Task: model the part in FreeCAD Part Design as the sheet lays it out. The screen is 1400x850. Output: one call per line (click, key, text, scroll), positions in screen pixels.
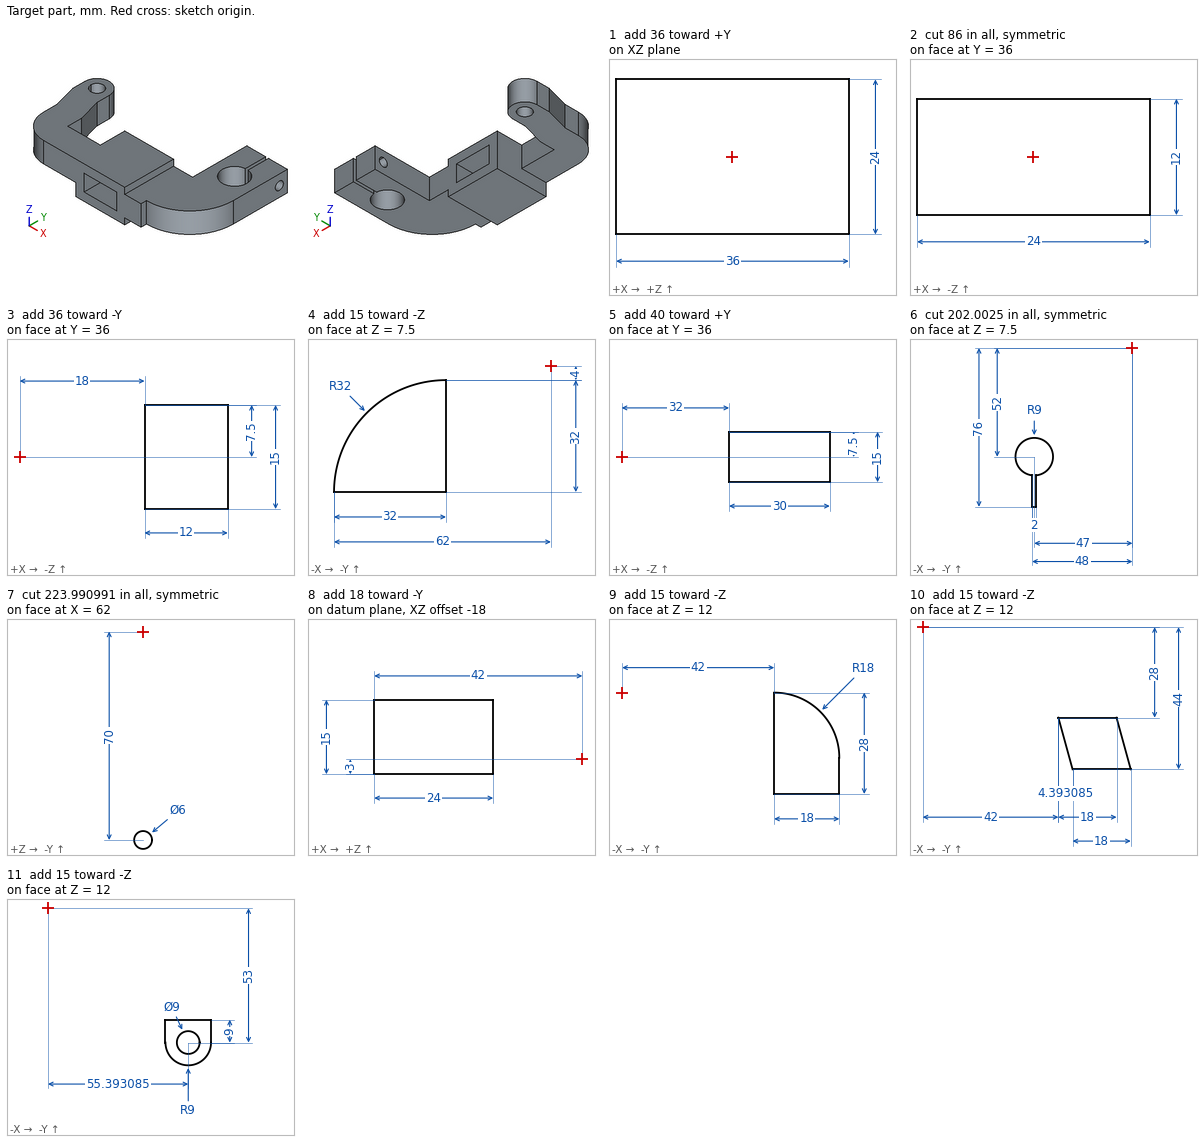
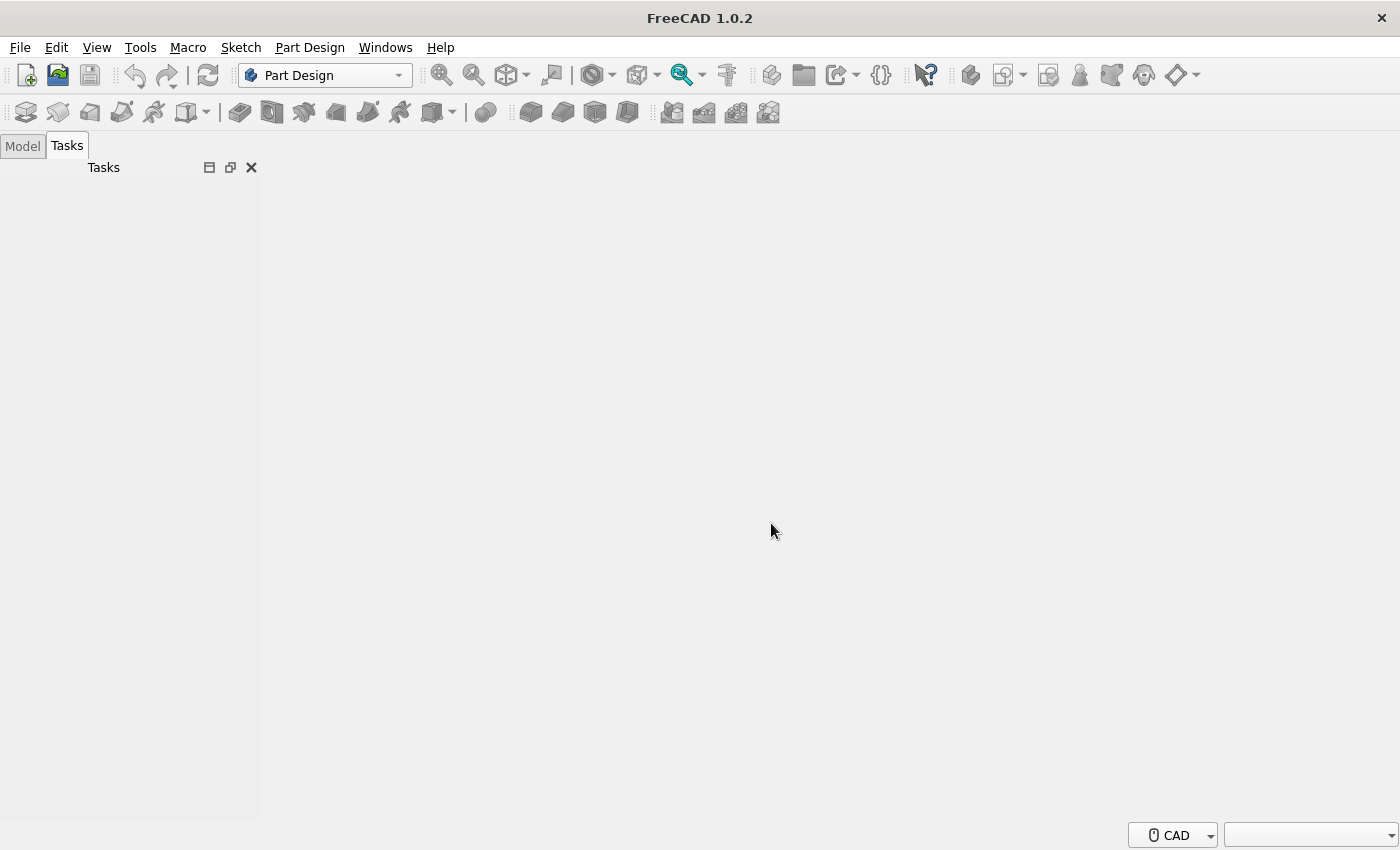
click(26, 76)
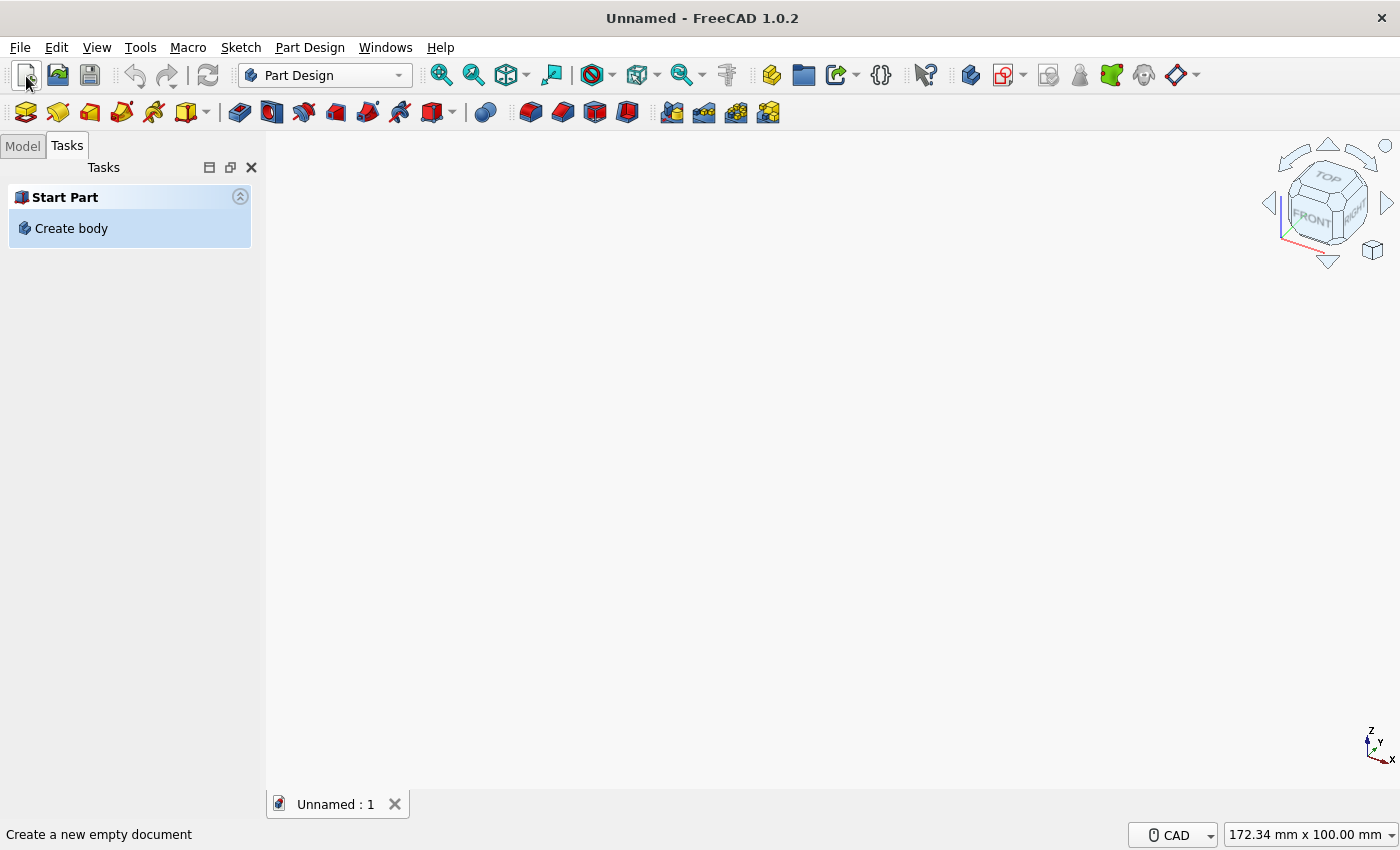
click(1004, 76)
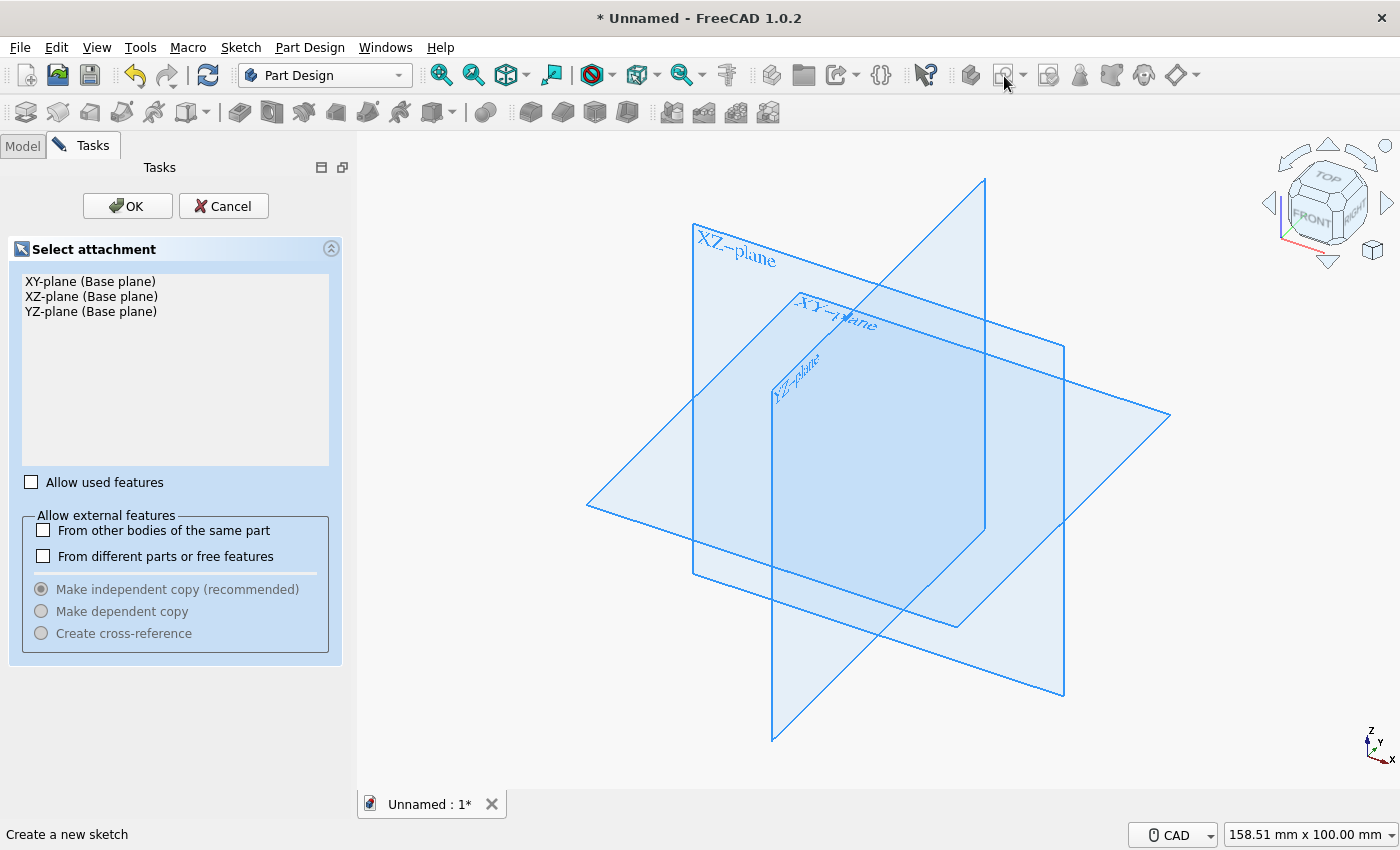
click(82, 296)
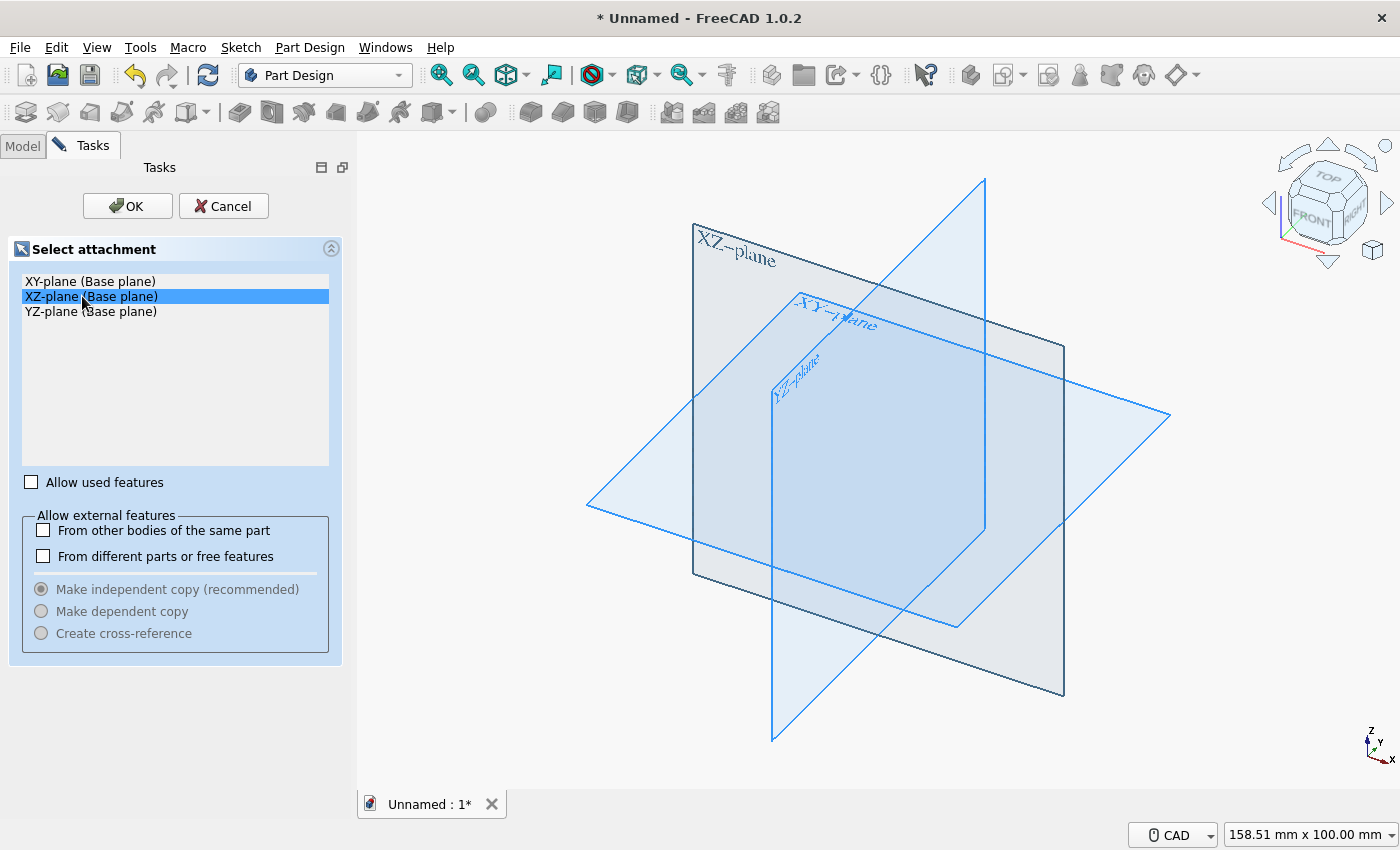
click(128, 206)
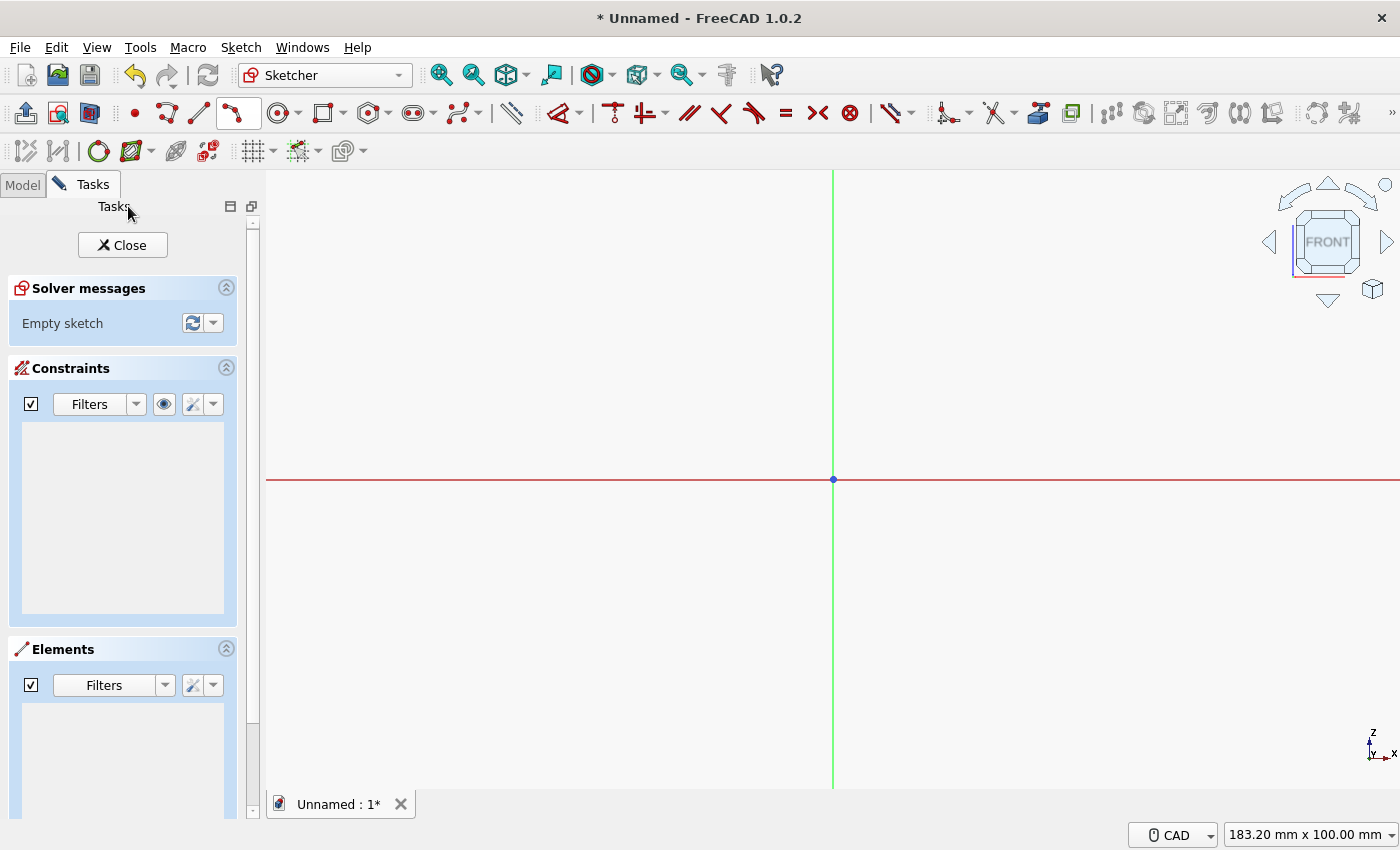
scroll(873, 480, up, 5)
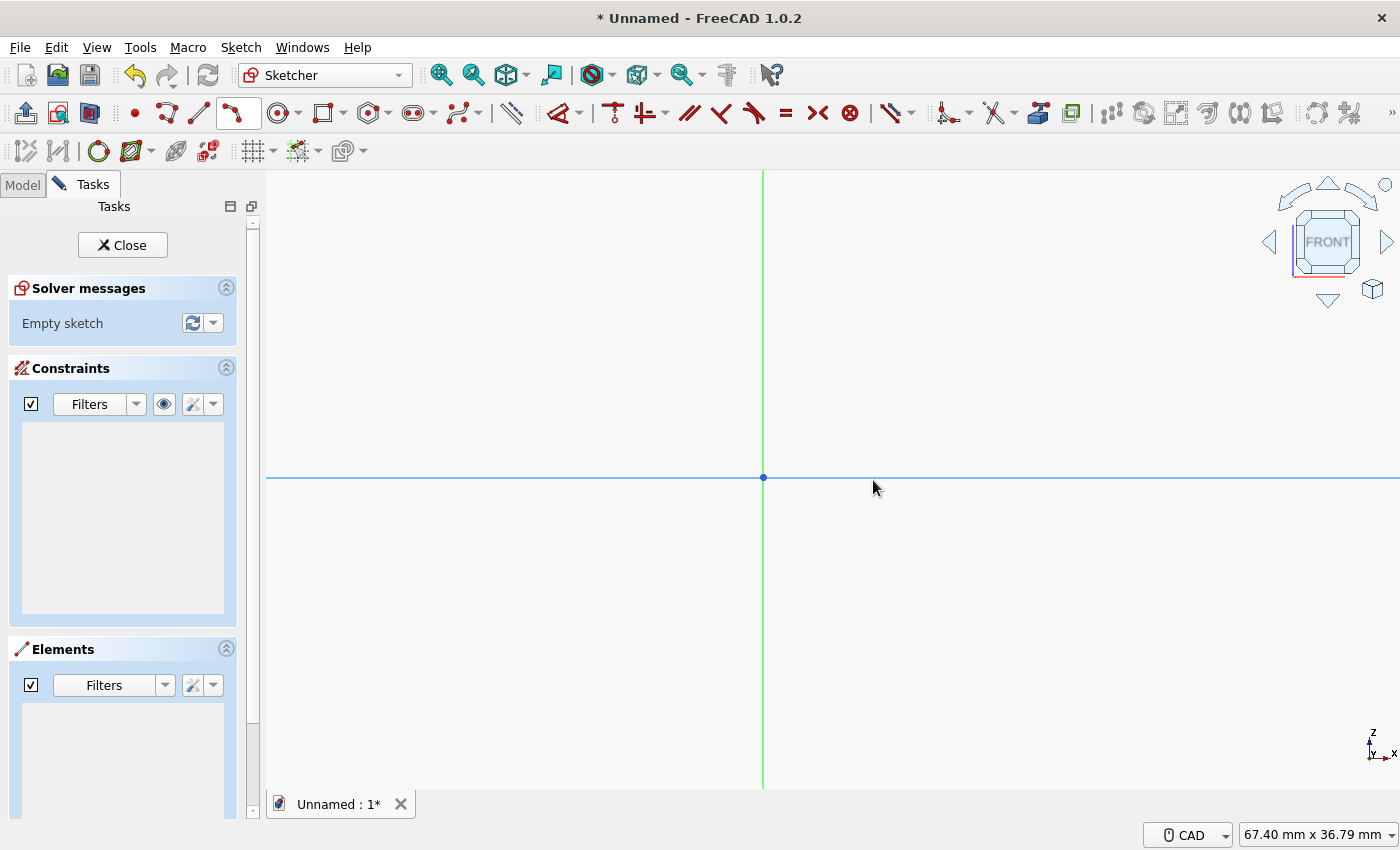
key(g)
key(v)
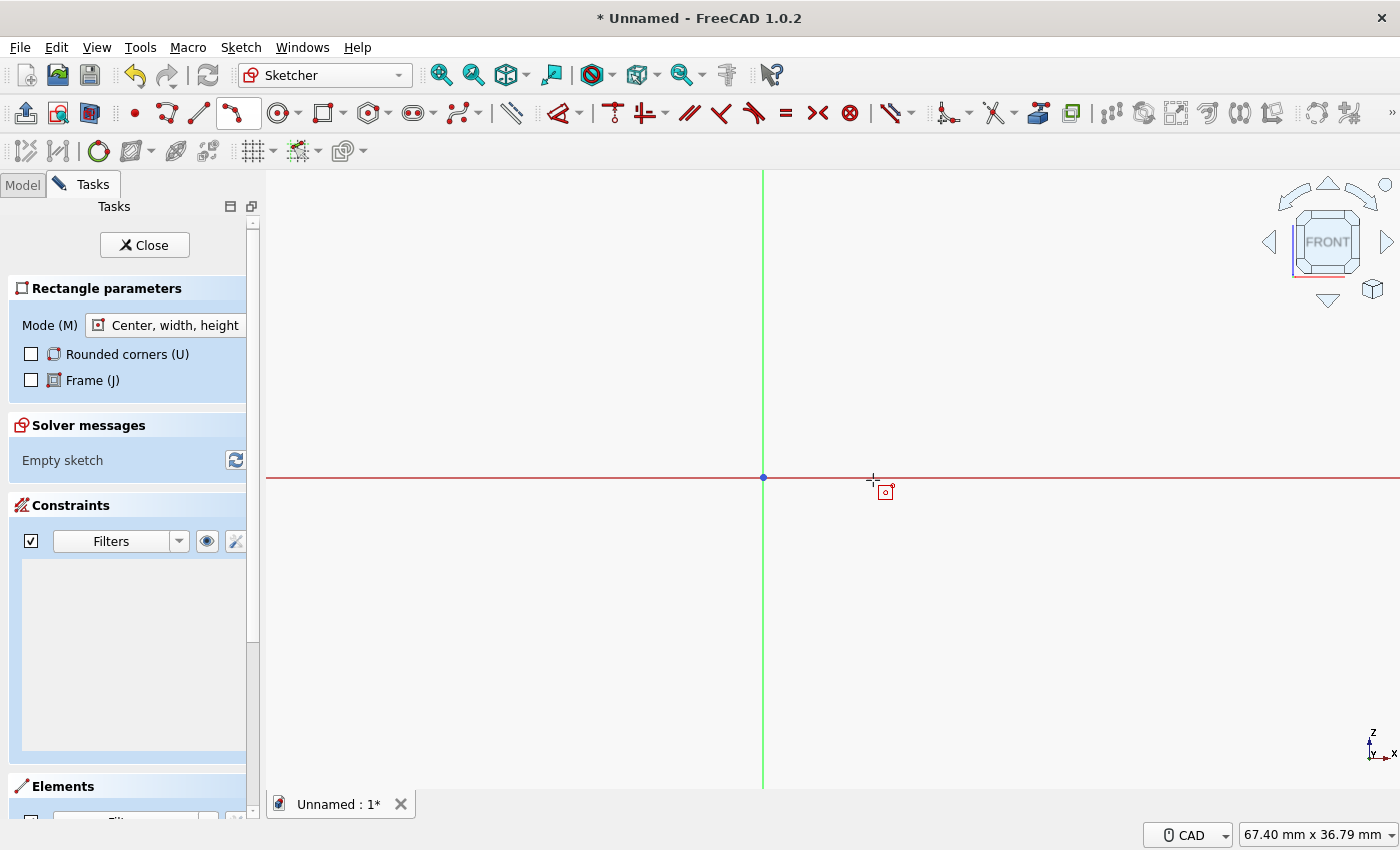
click(763, 478)
click(1066, 276)
key(Escape)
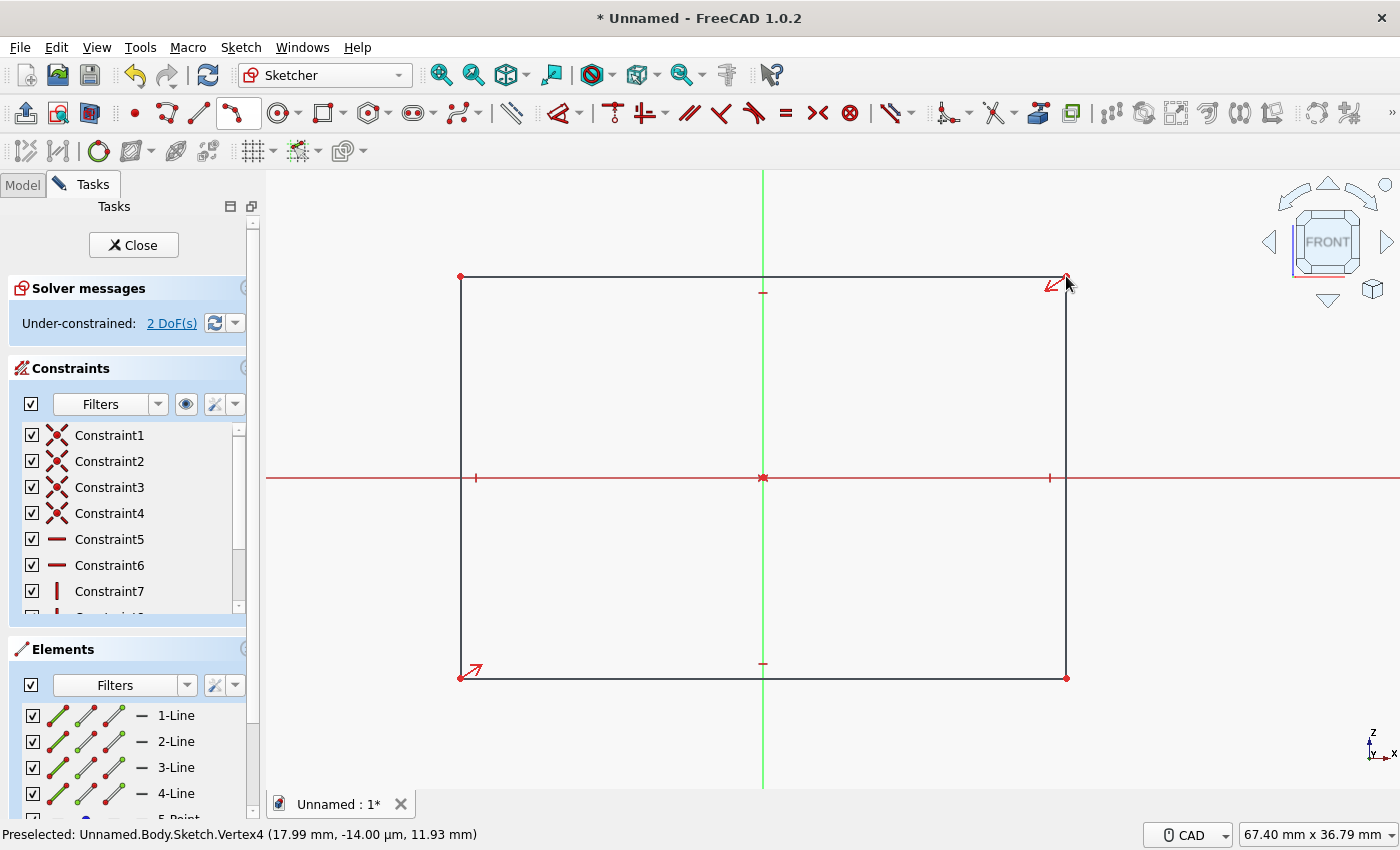
key(d)